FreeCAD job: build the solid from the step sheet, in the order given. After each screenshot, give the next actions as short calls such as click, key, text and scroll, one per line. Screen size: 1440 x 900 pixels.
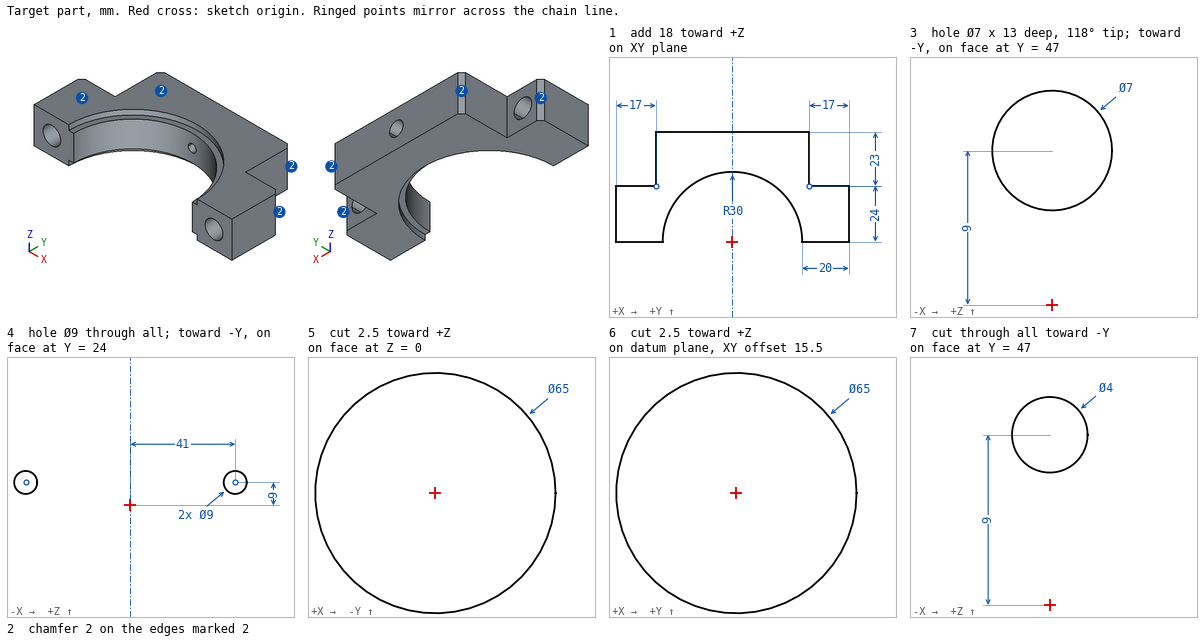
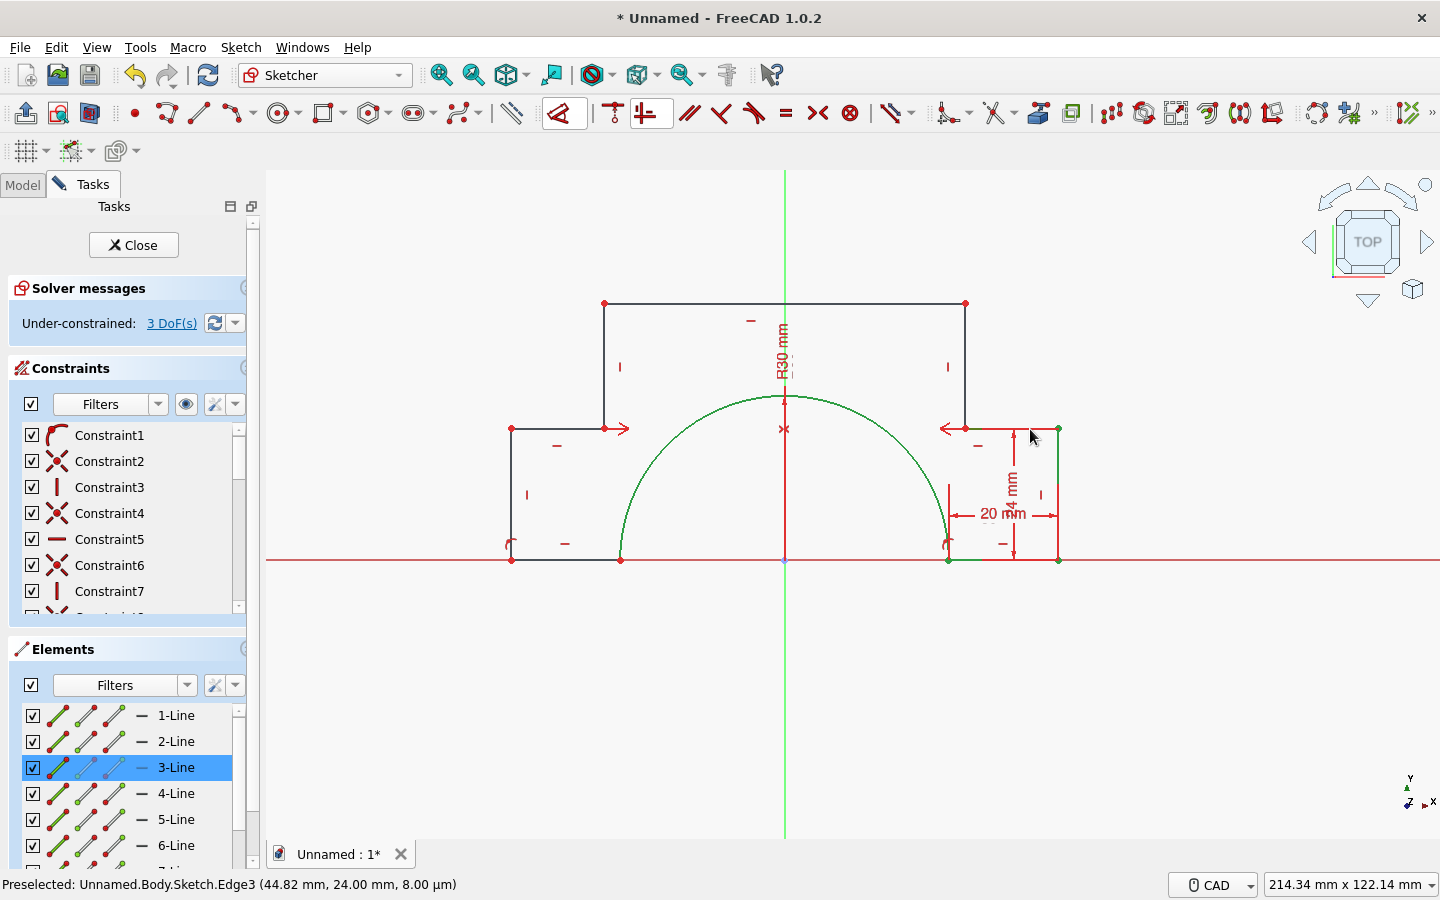
key(l)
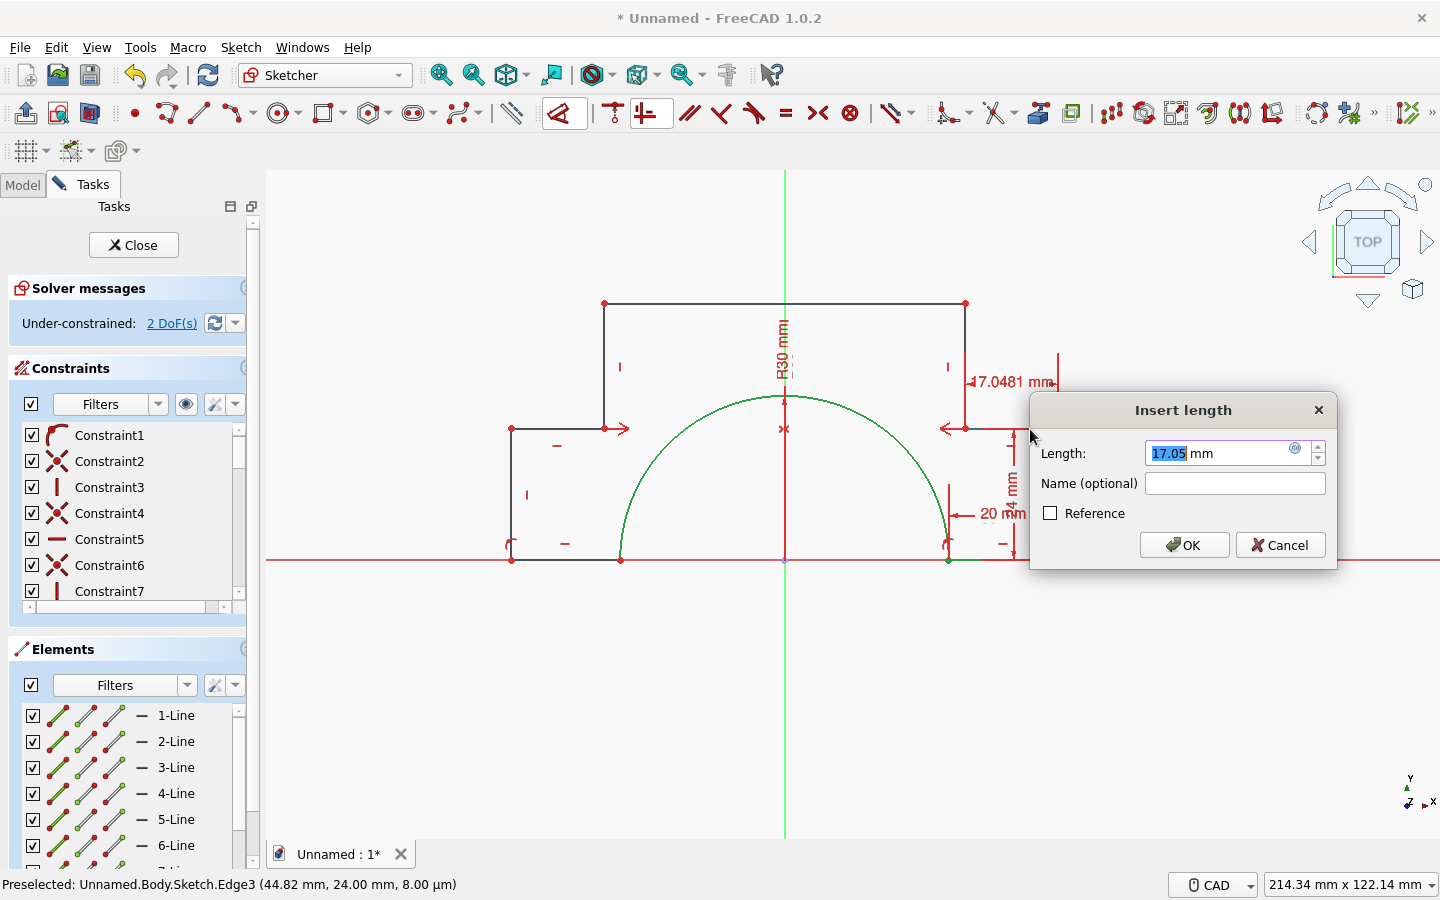
text(17)
key(Return)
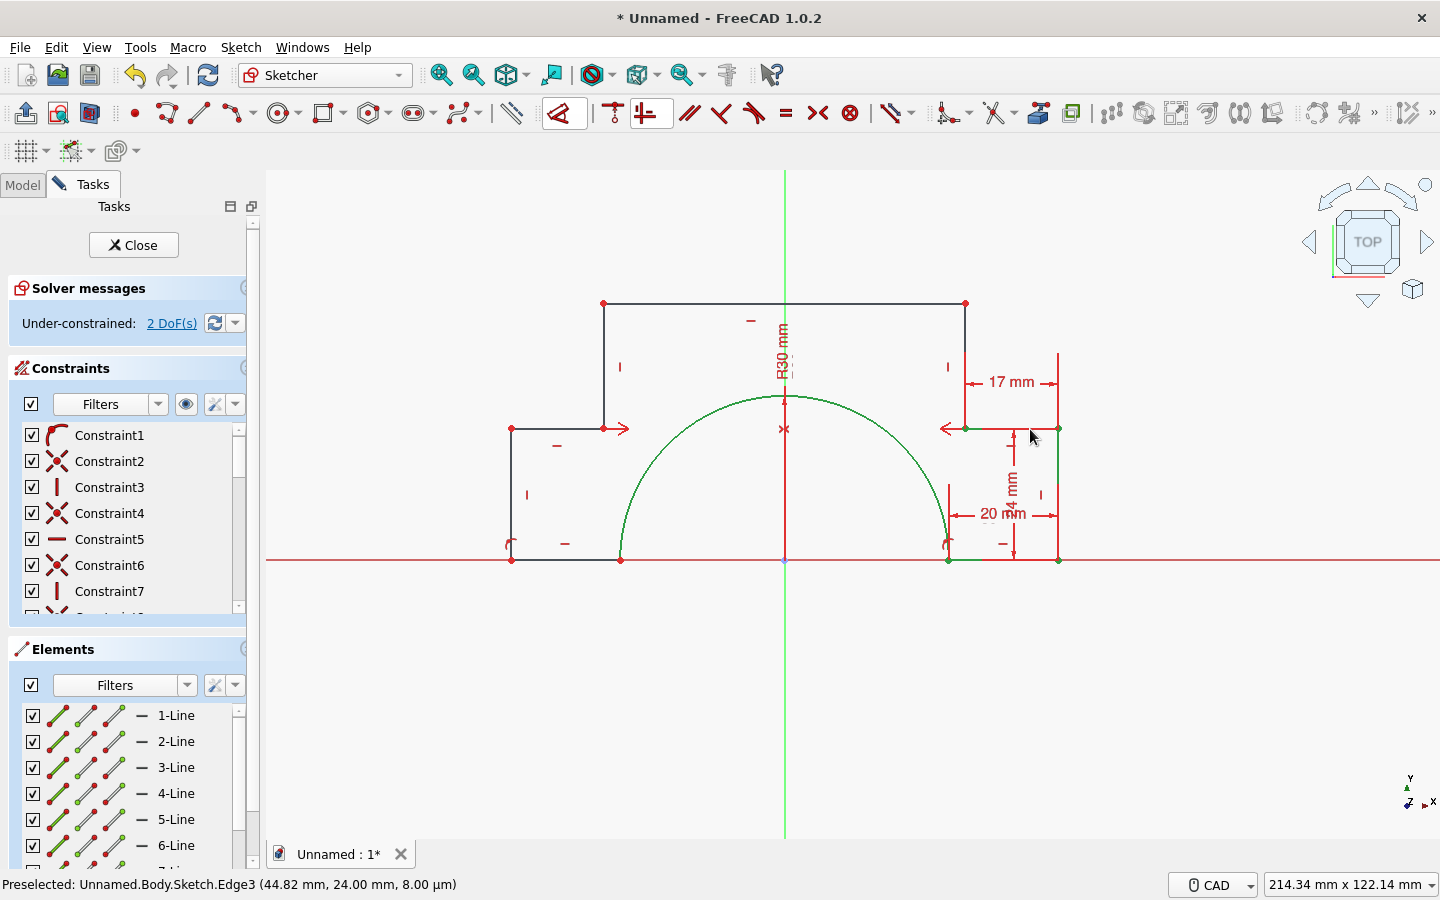
click(965, 391)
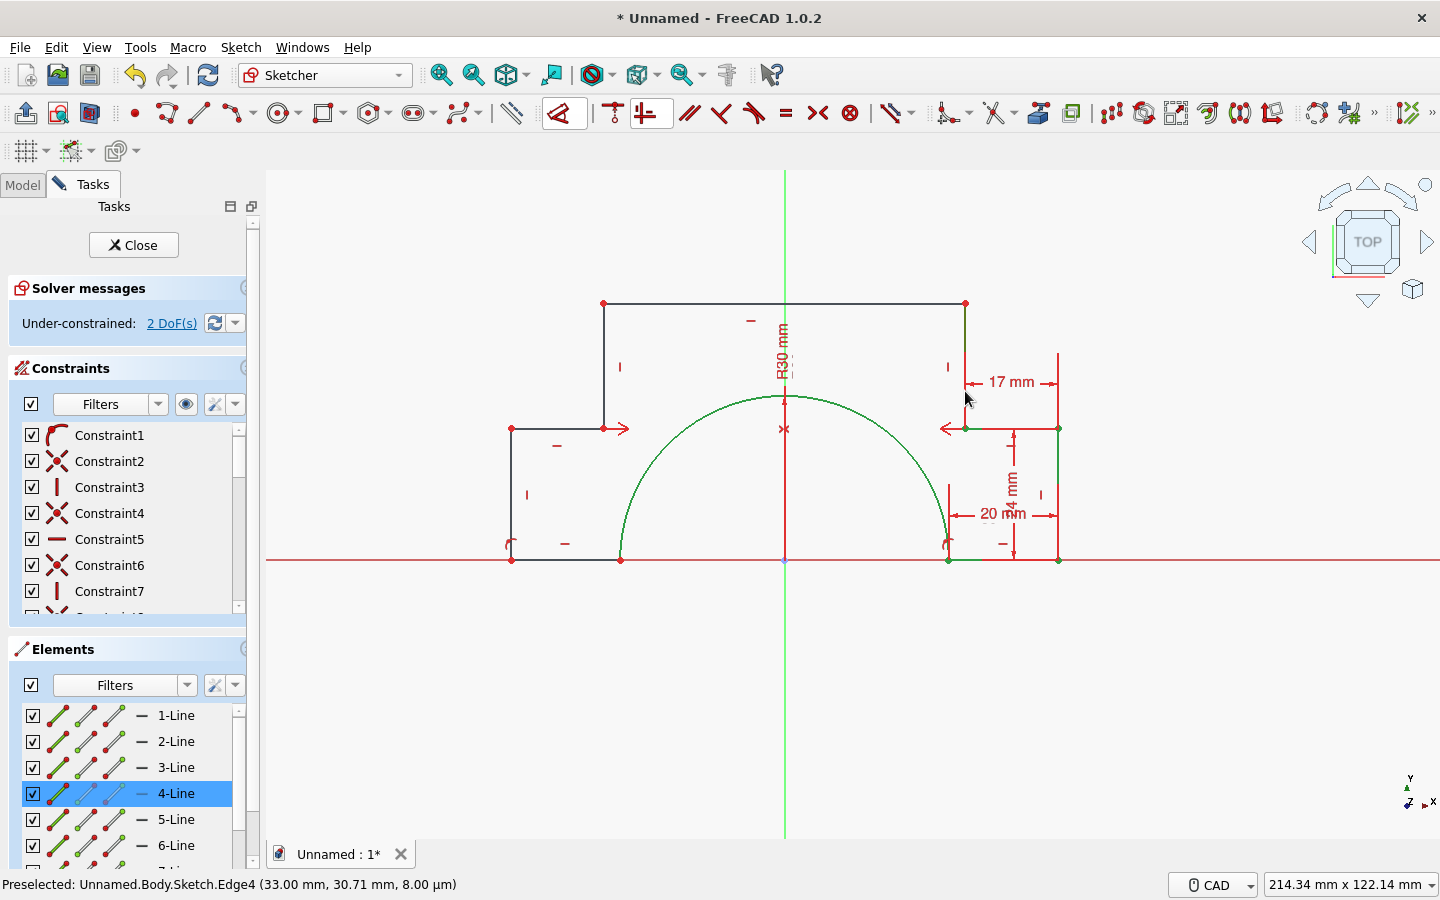
key(i)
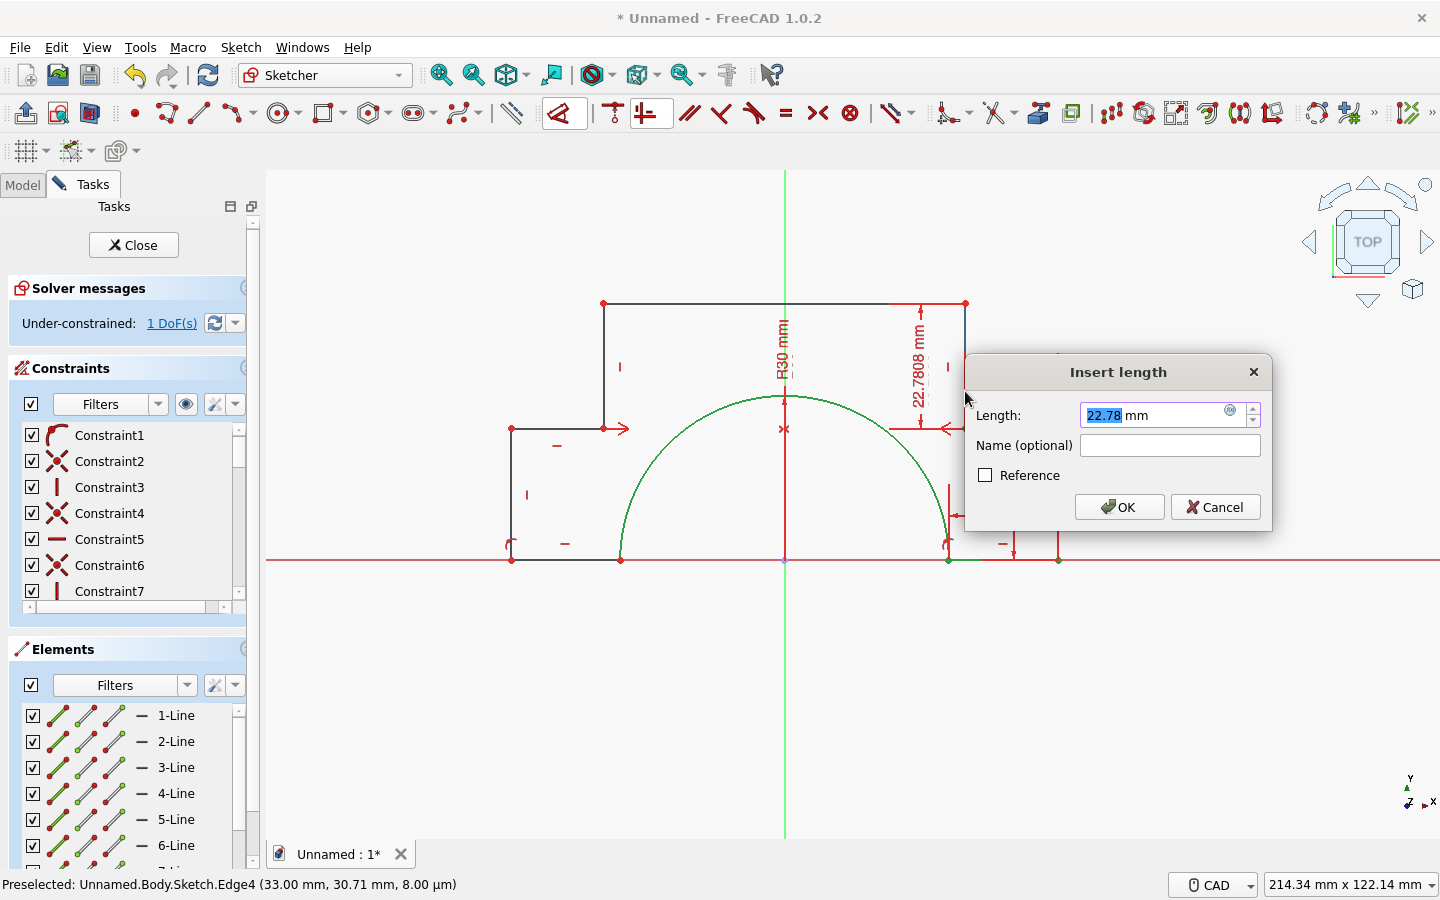
text(23)
key(Return)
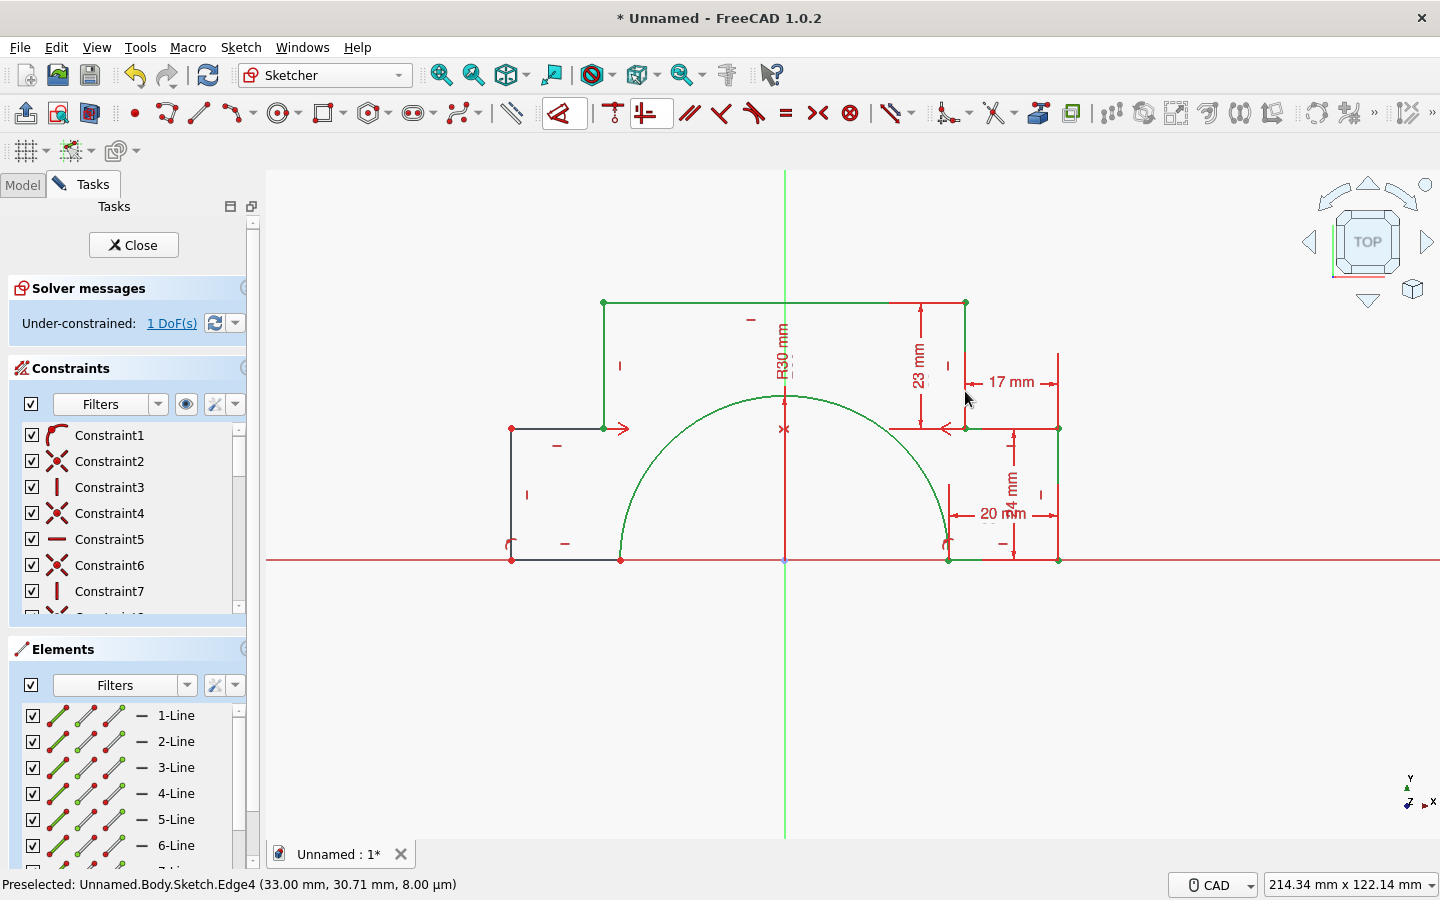
click(576, 429)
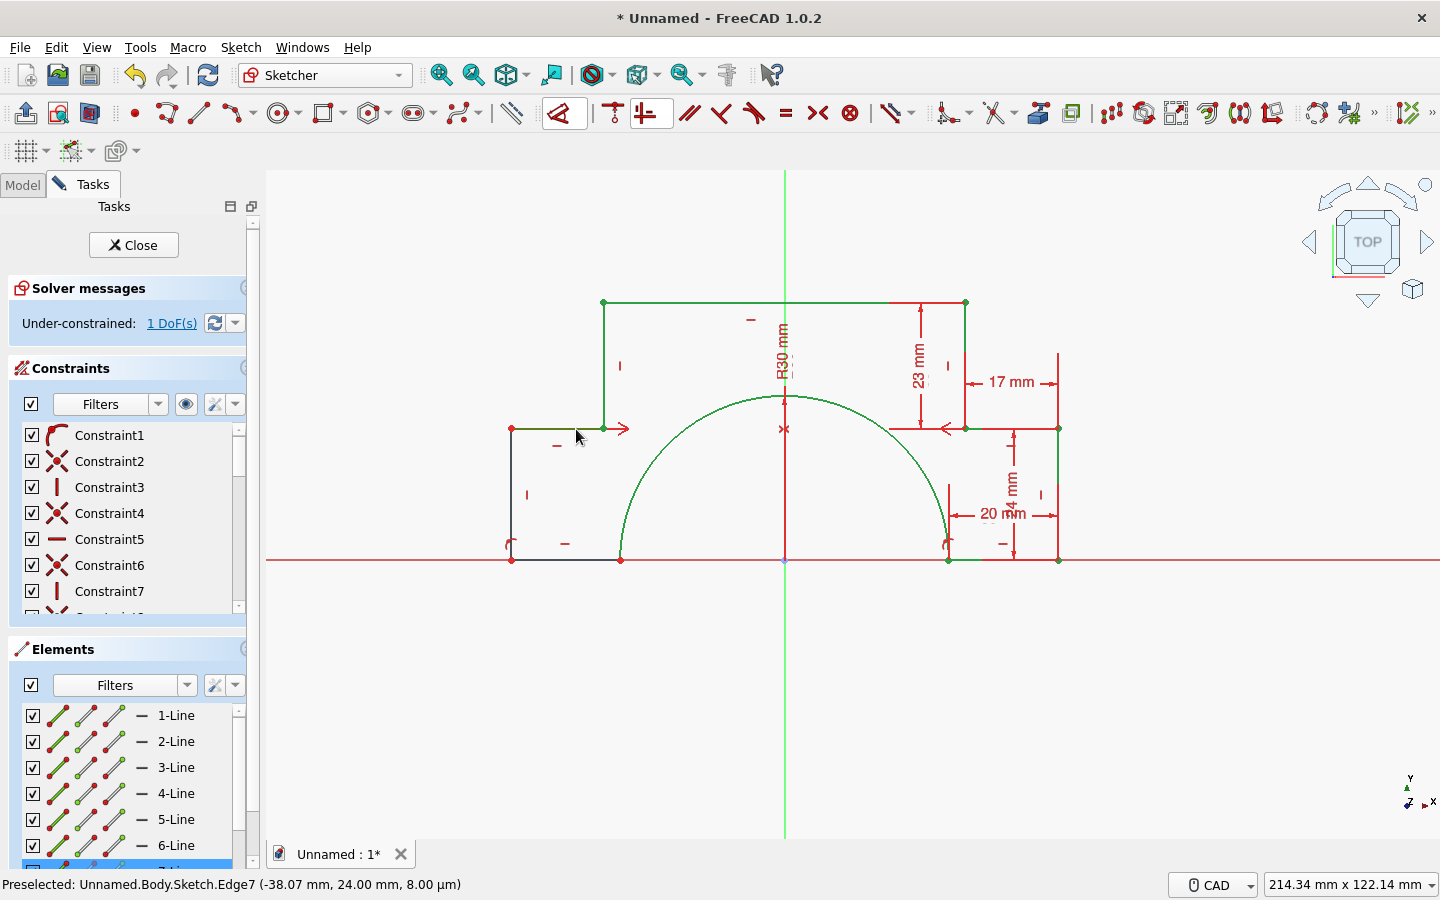
key(l)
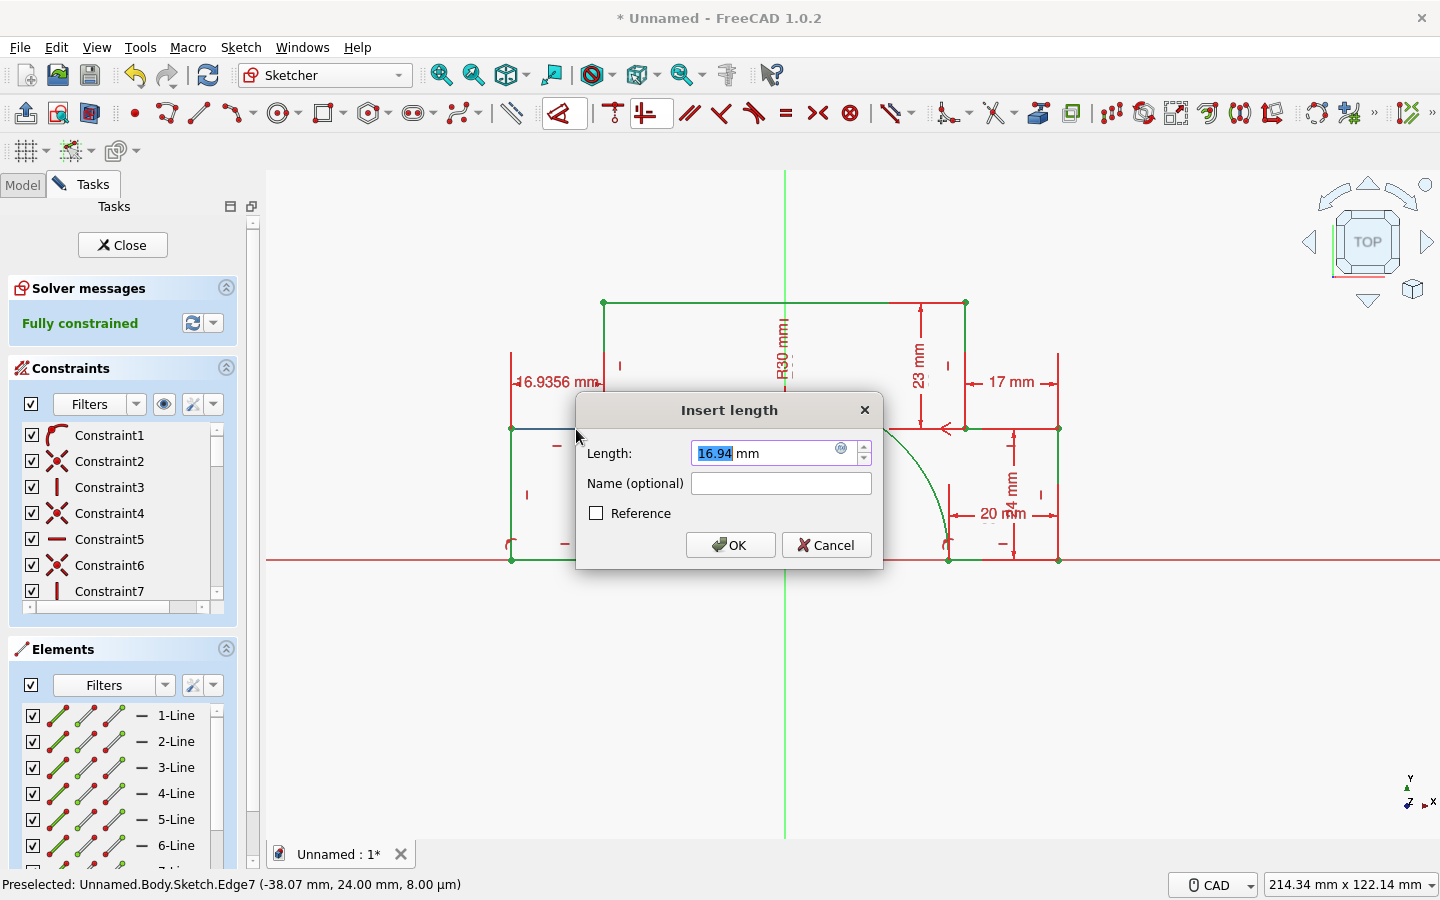
text(17)
key(Return)